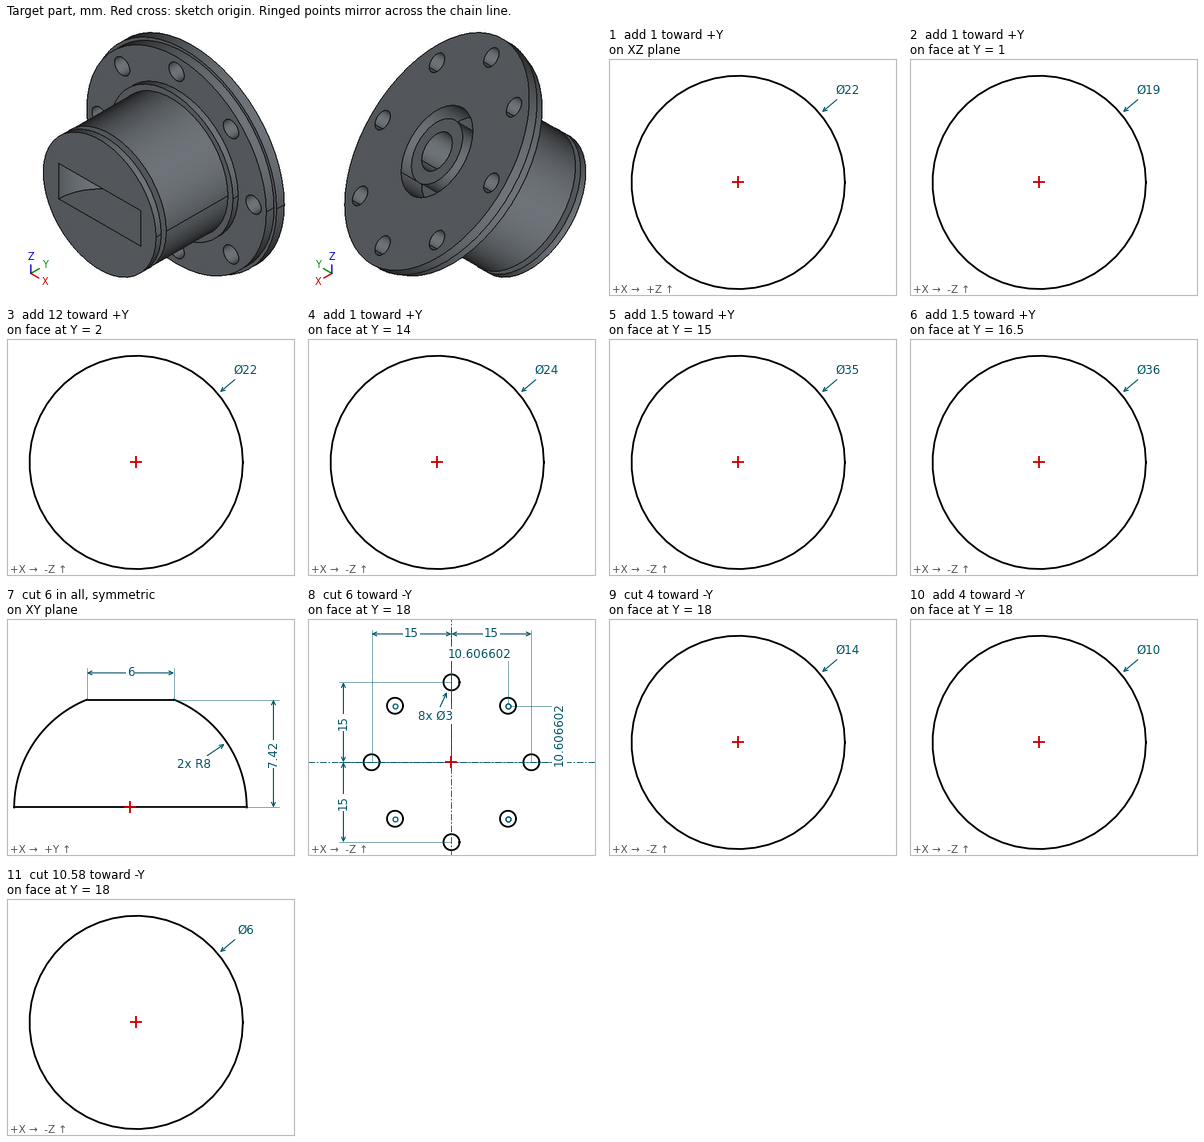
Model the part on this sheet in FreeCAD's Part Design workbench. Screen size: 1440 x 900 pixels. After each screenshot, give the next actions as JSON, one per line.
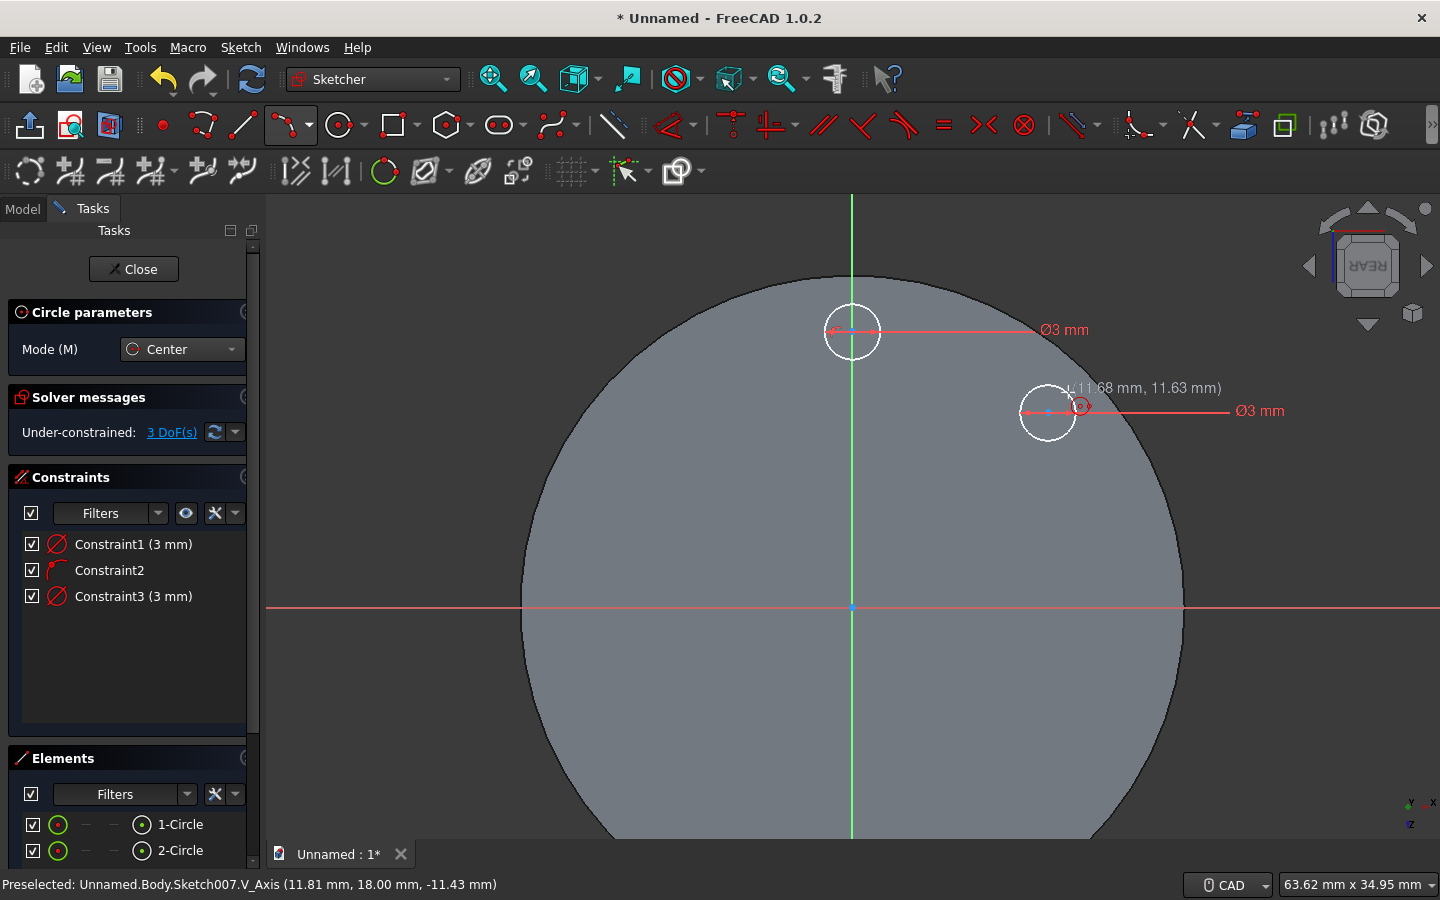
{"action": "left_click", "coordinate": [1129, 608]}
{"action": "mouse_move", "coordinate": [1149, 588]}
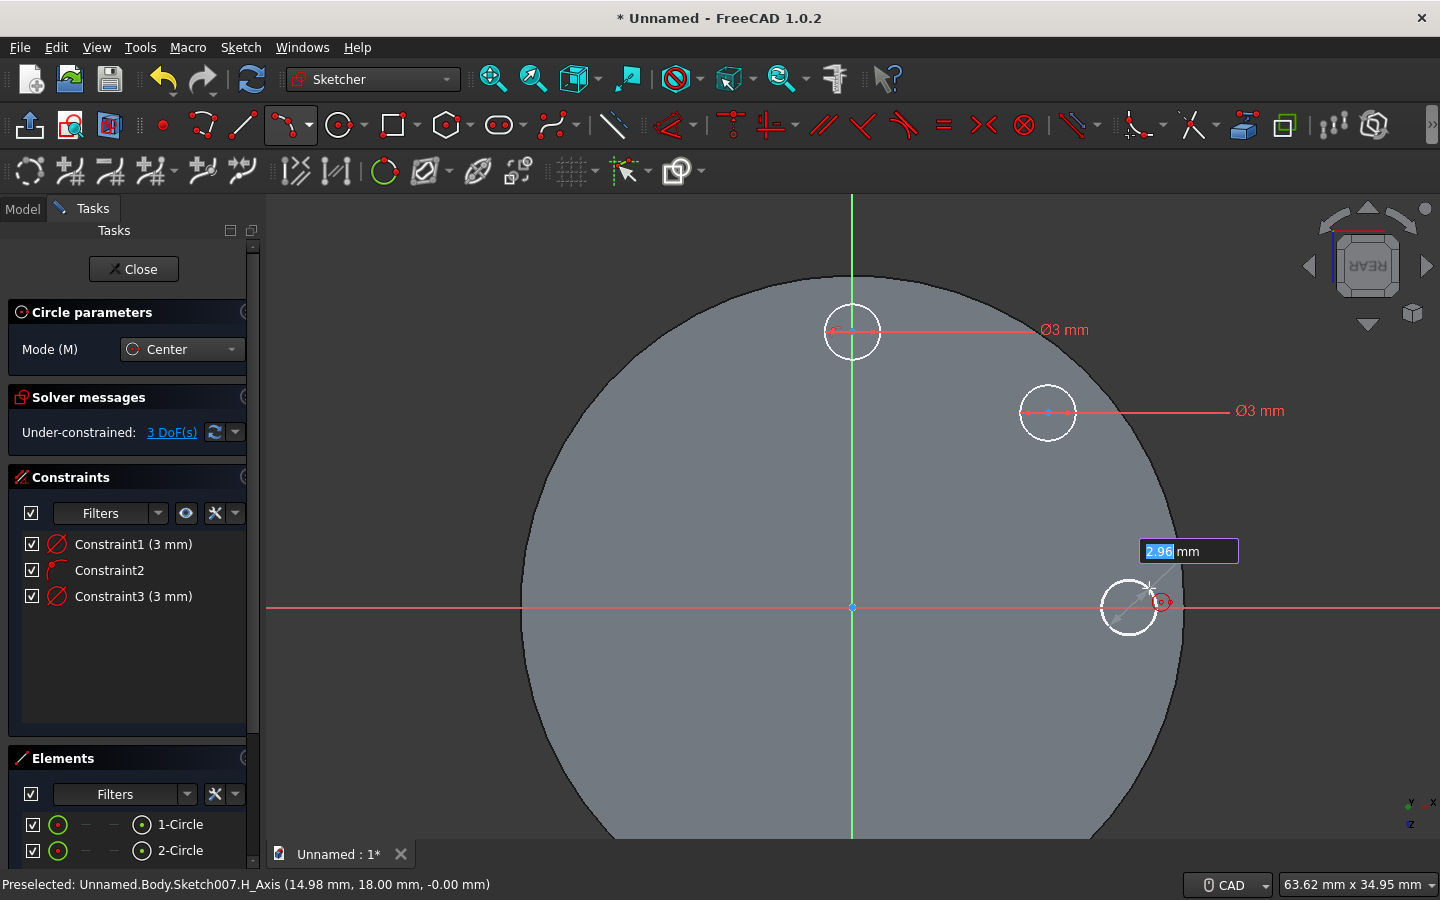
{"action": "type", "text": "3"}
{"action": "key", "text": "Return"}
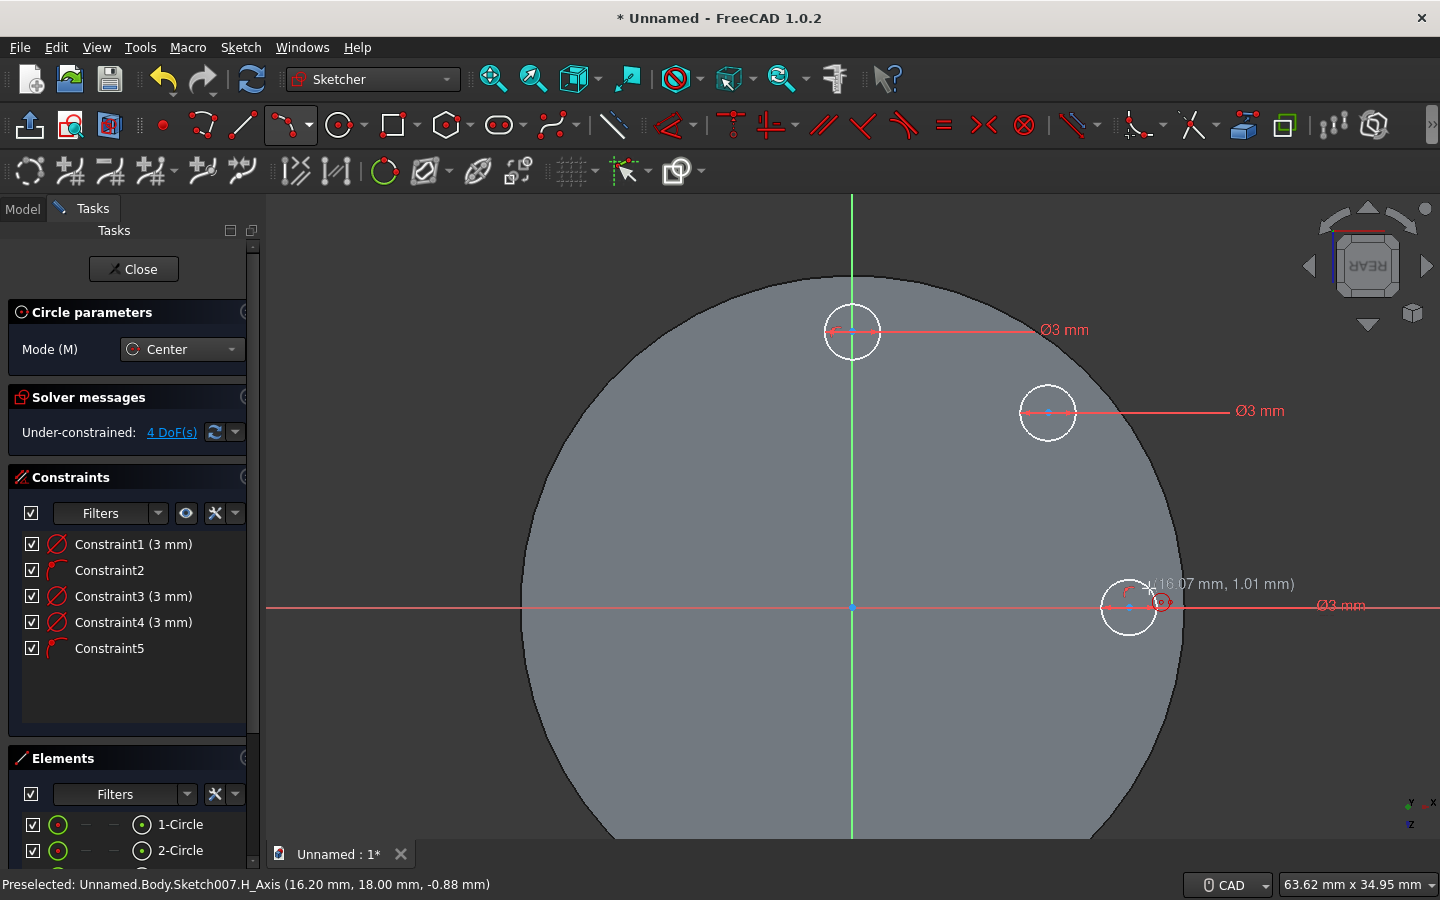
{"action": "left_click", "coordinate": [1048, 803]}
{"action": "mouse_move", "coordinate": [1068, 784]}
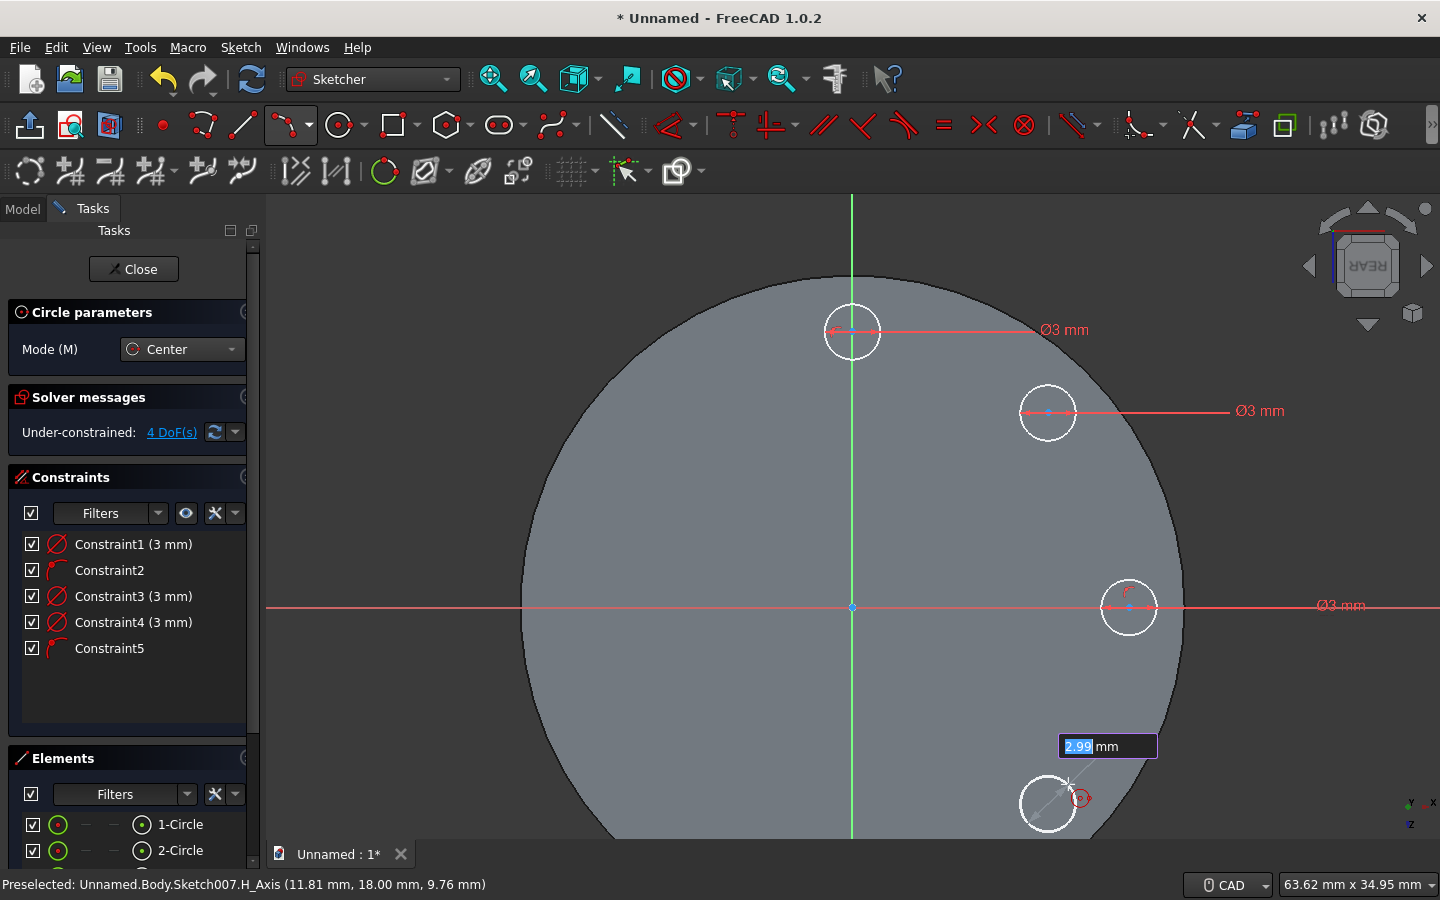
{"action": "type", "text": "3"}
{"action": "key", "text": "Return"}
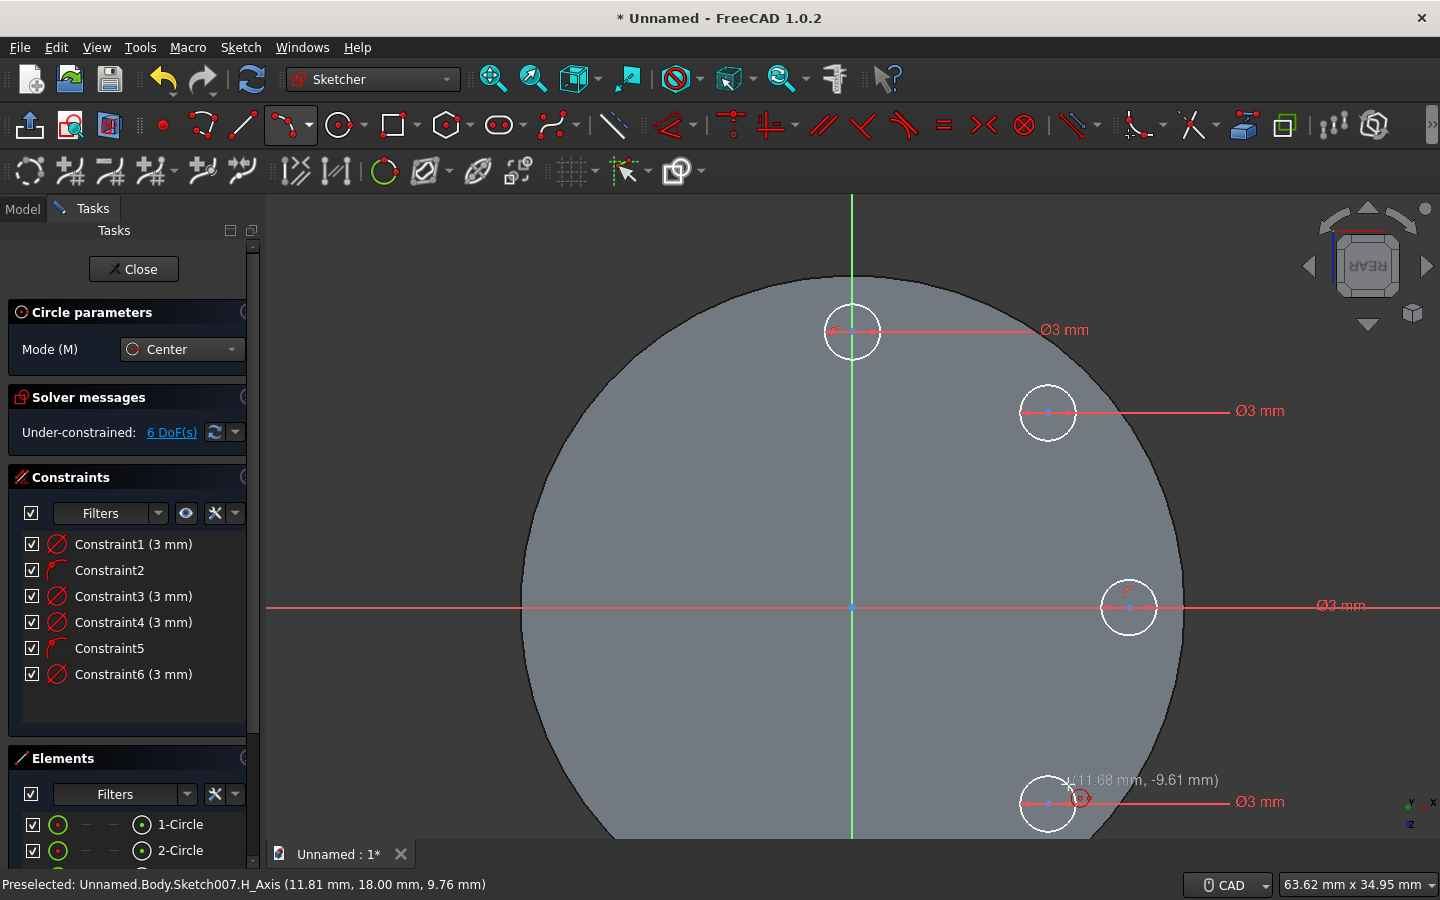
{"action": "scroll", "coordinate": [646, 331], "scroll_direction": "down", "scroll_amount": 2}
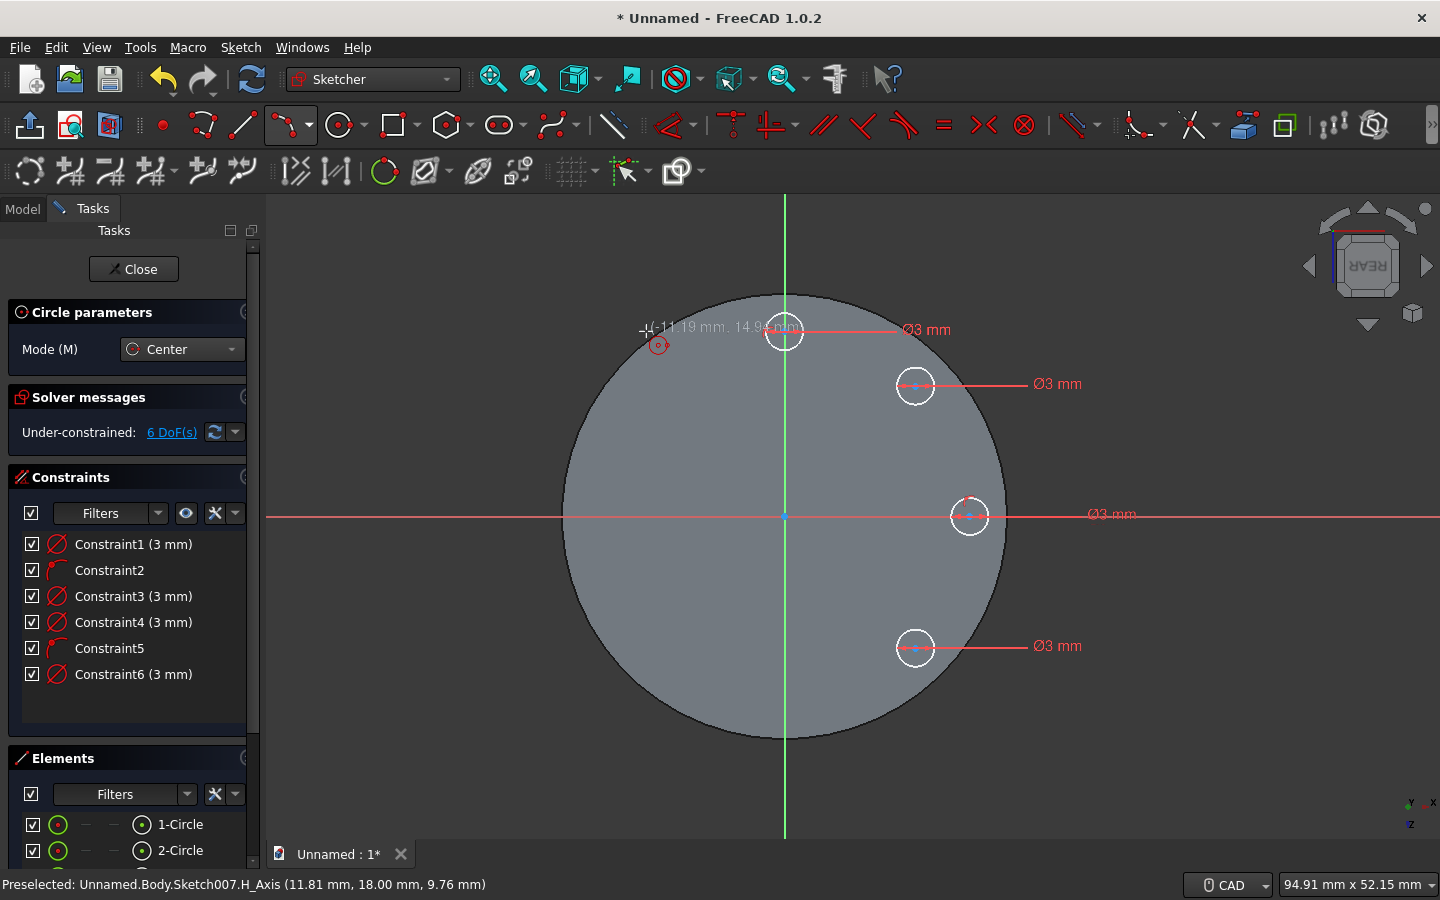
{"action": "scroll", "coordinate": [785, 702], "scroll_direction": "up", "scroll_amount": 2}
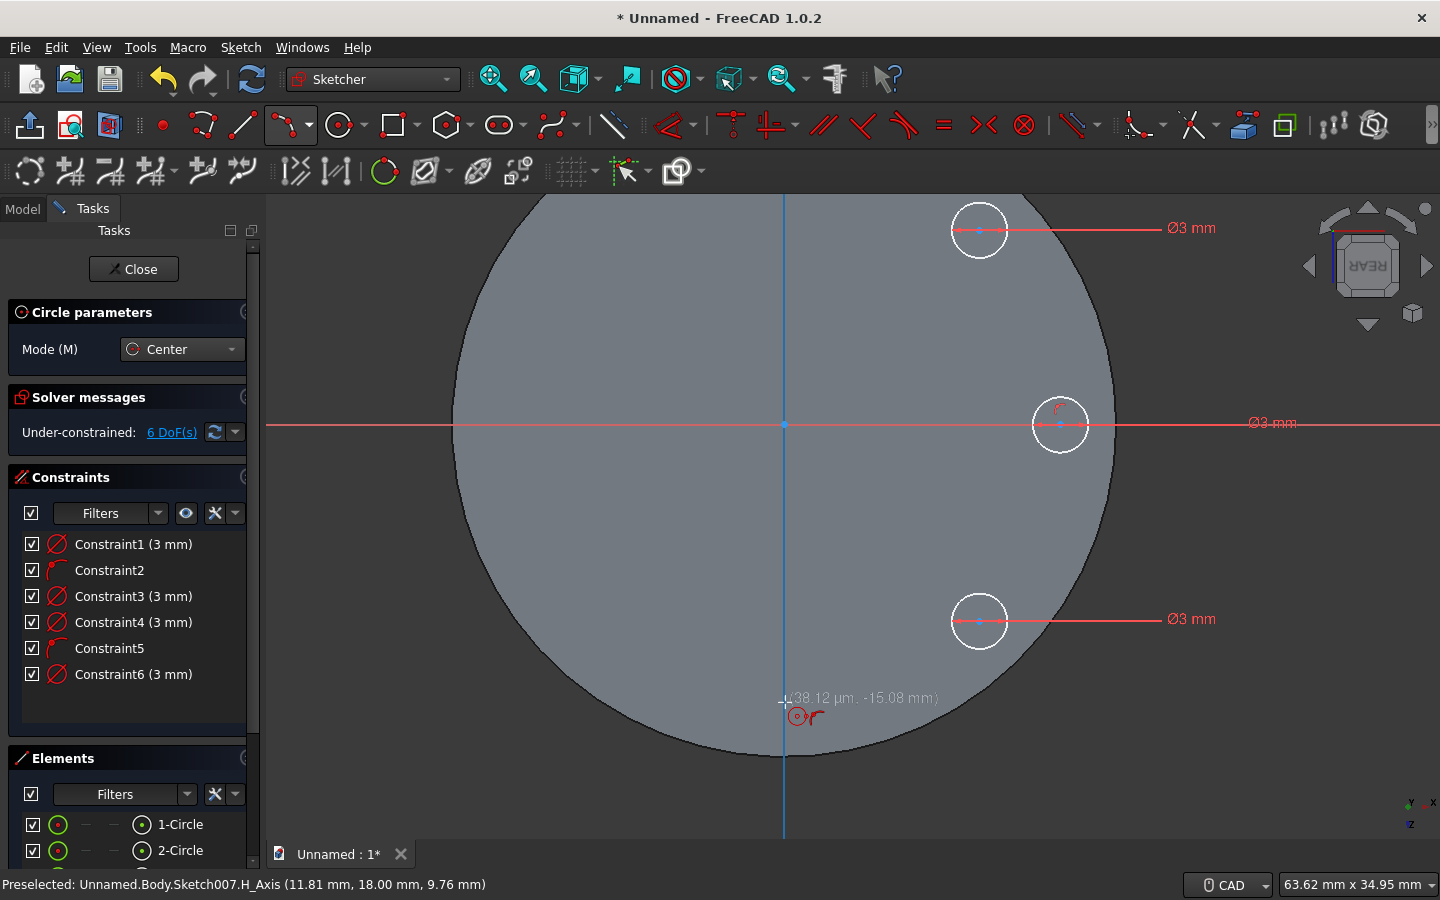
{"action": "left_click", "coordinate": [784, 702]}
{"action": "mouse_move", "coordinate": [804, 682]}